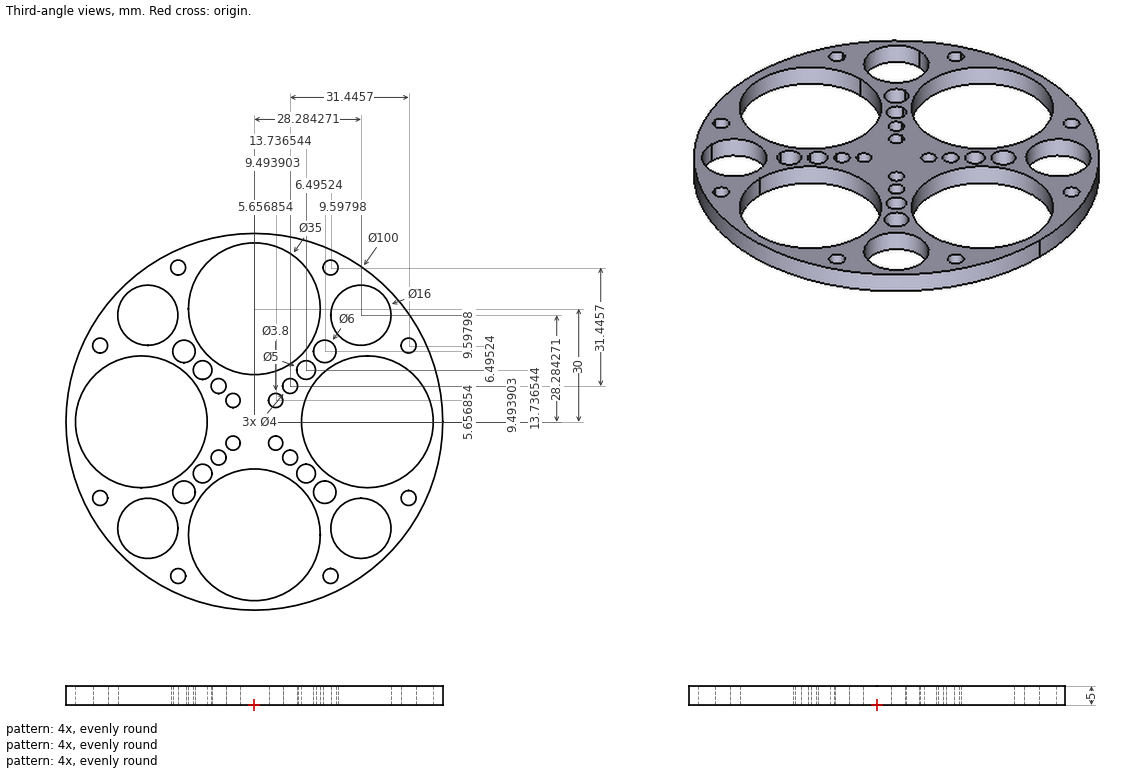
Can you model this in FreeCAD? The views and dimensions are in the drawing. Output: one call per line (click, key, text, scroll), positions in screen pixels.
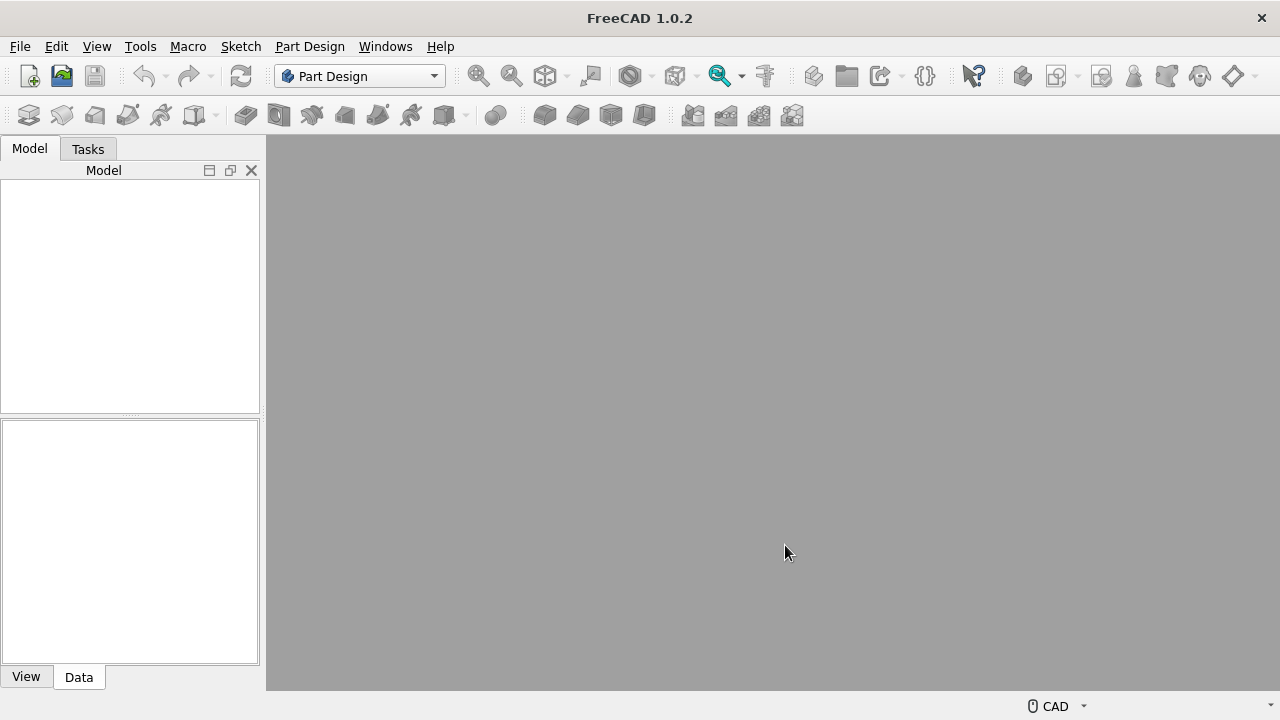
click(29, 76)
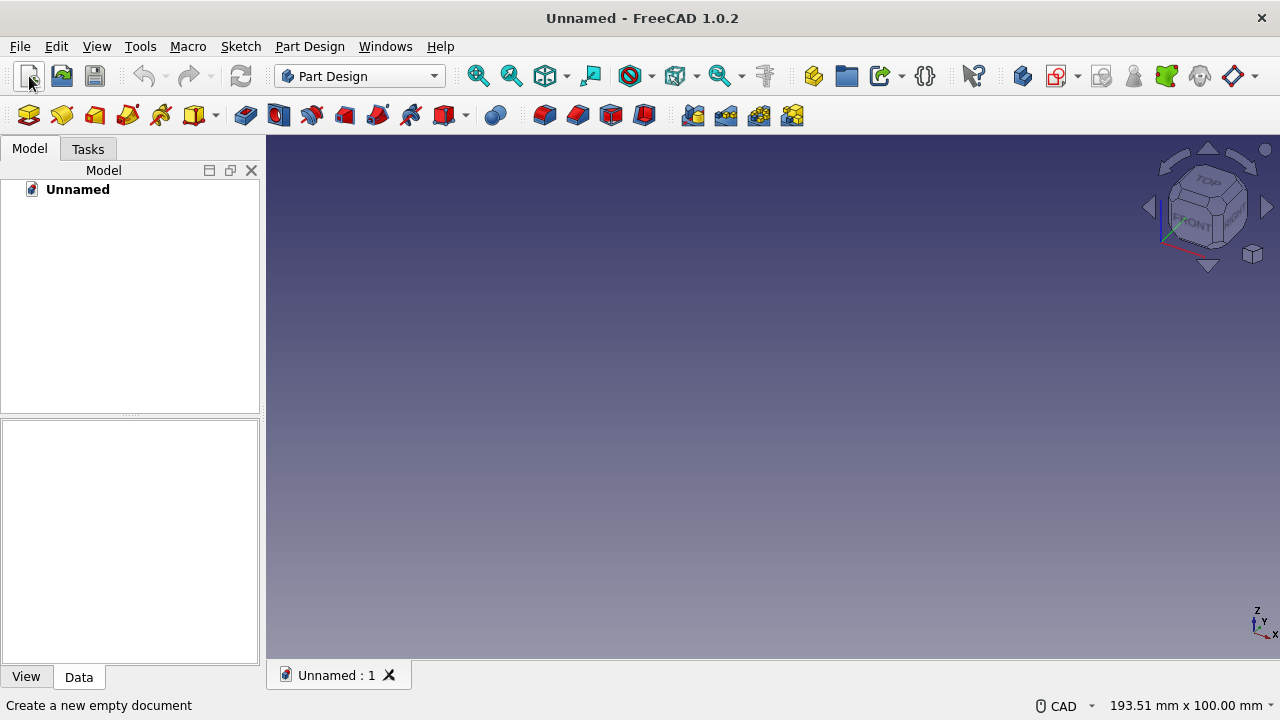
click(1056, 76)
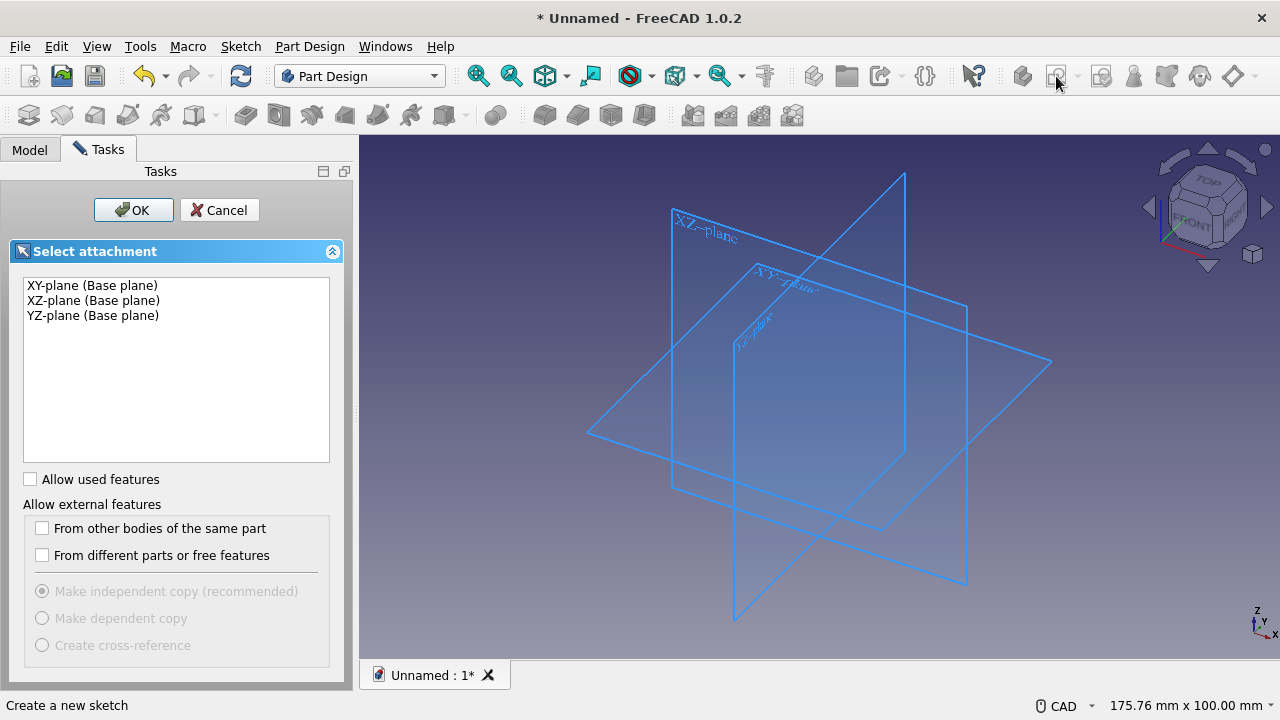
click(84, 286)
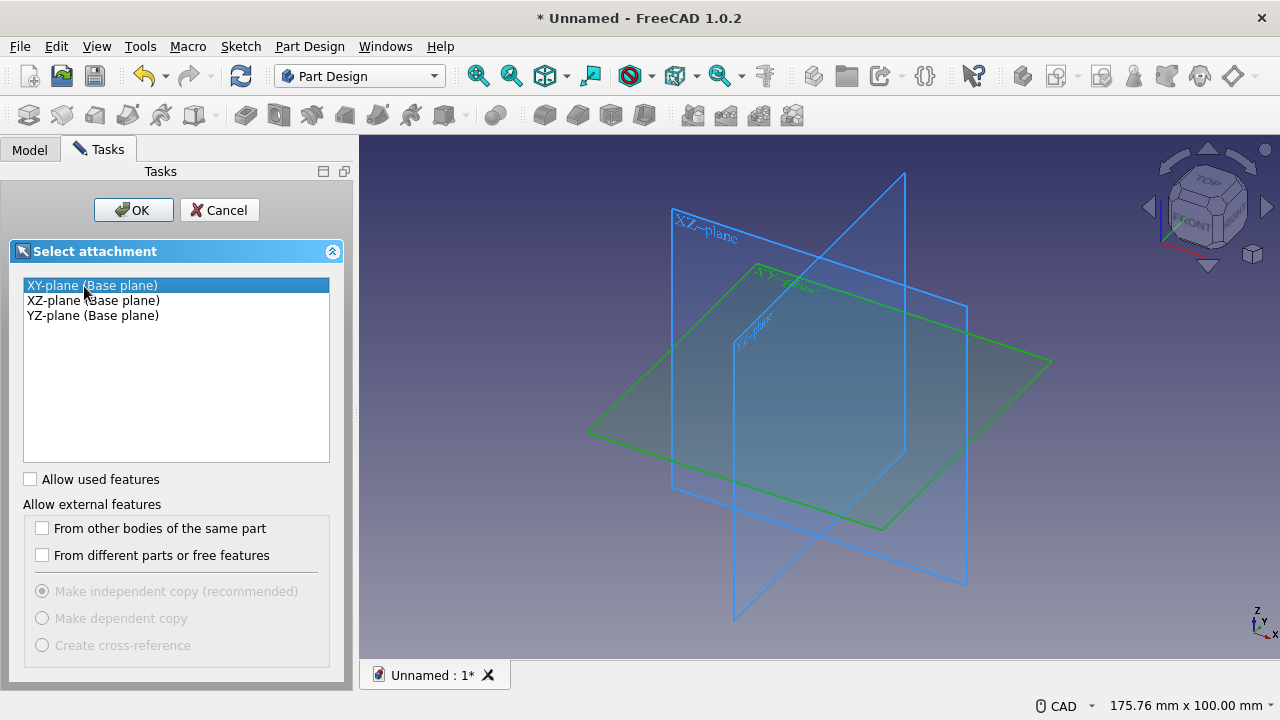
click(134, 210)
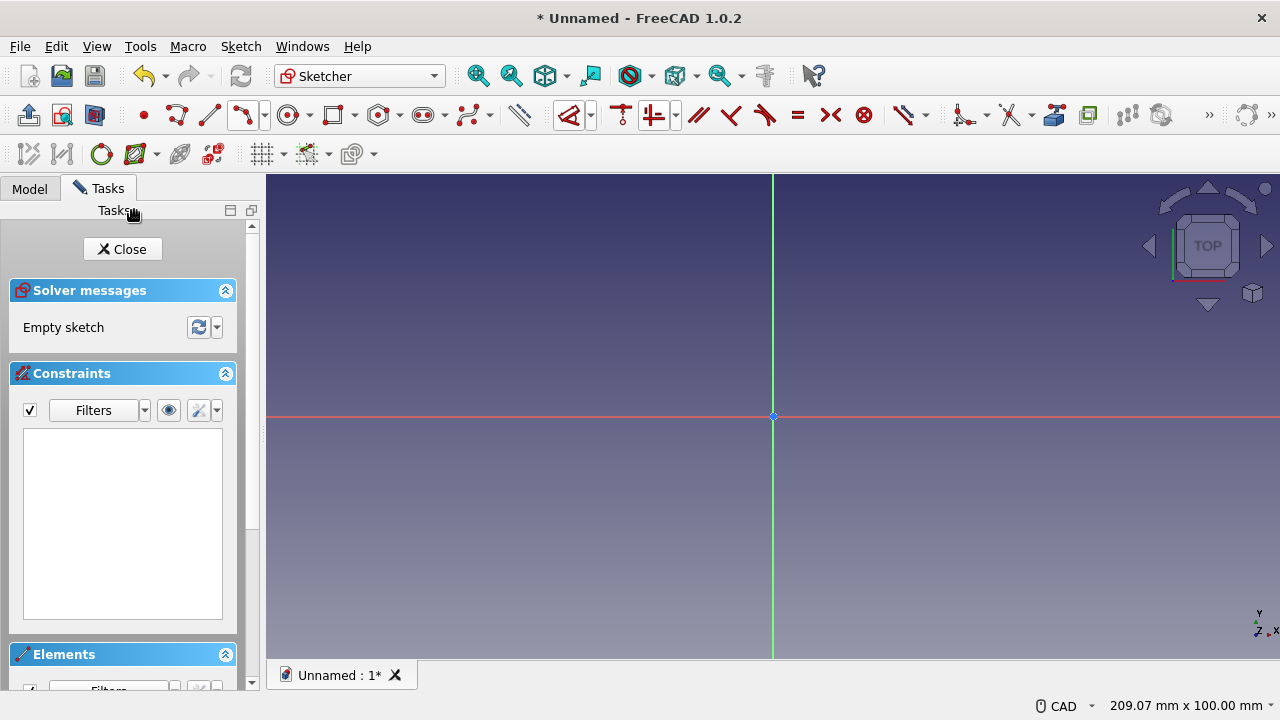
scroll(565, 416, down, 2)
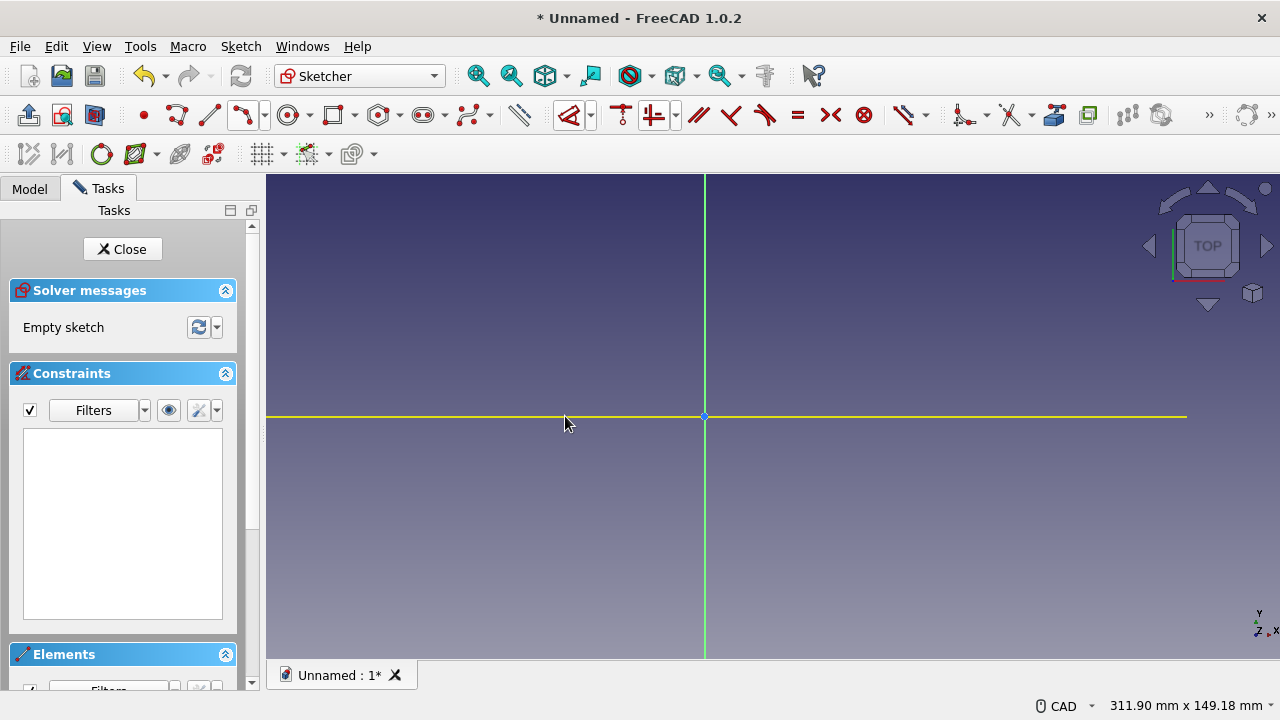
click(288, 116)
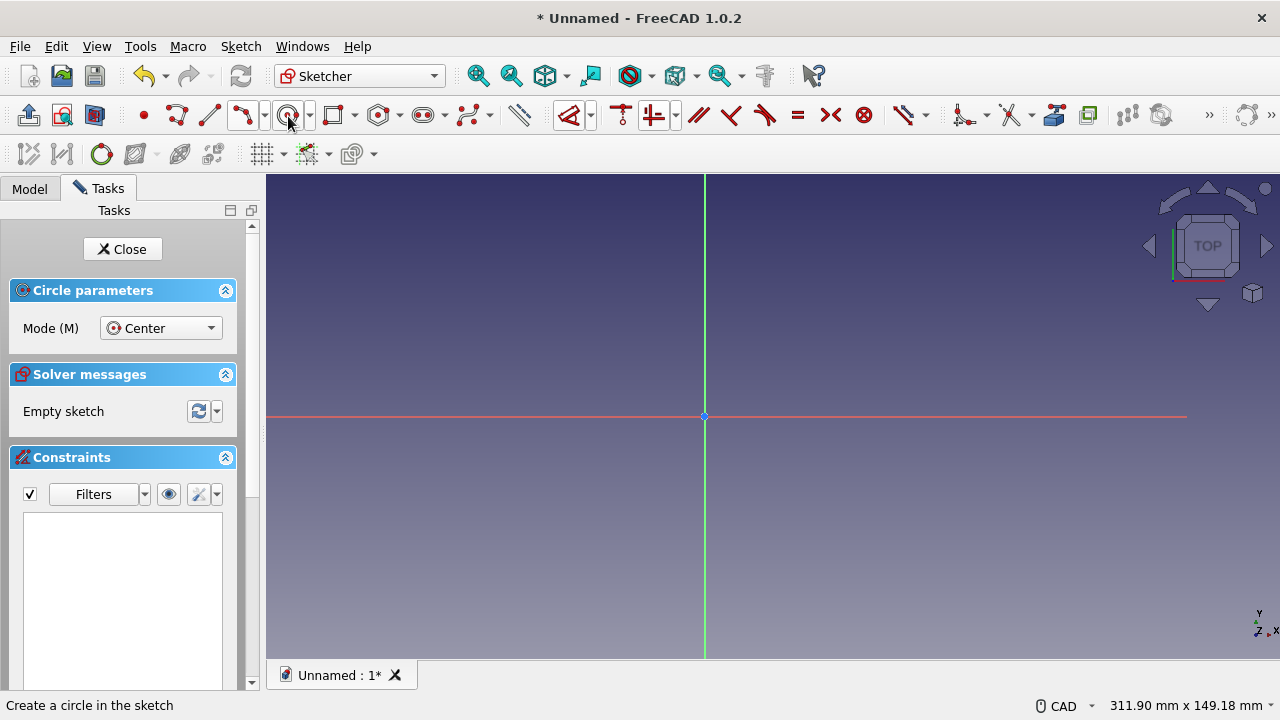
click(705, 416)
click(819, 302)
key(Escape)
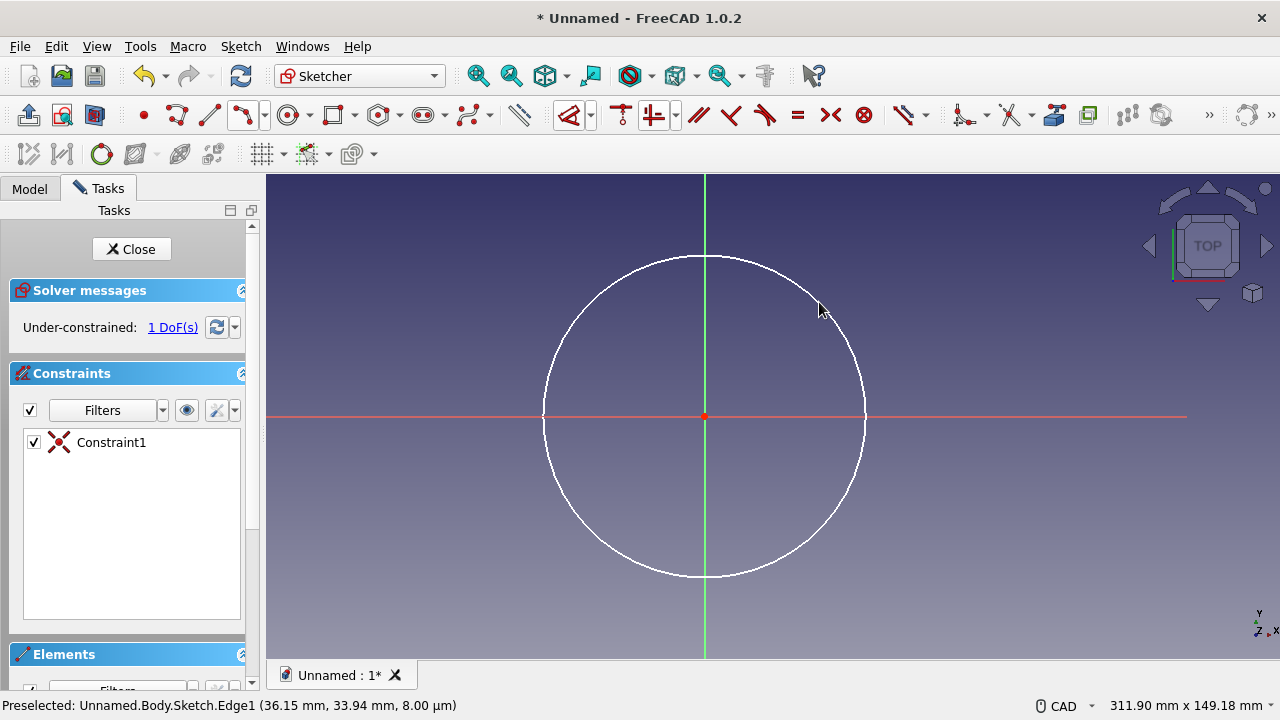
click(568, 116)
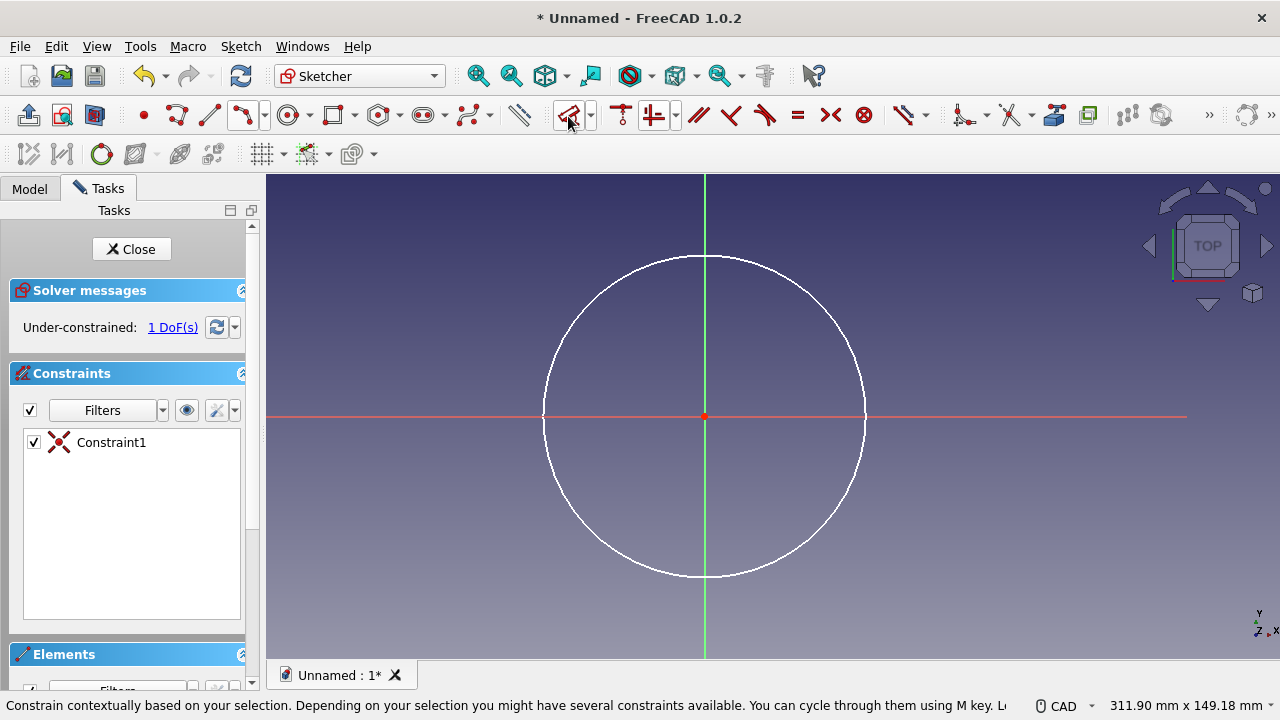
click(818, 302)
click(841, 279)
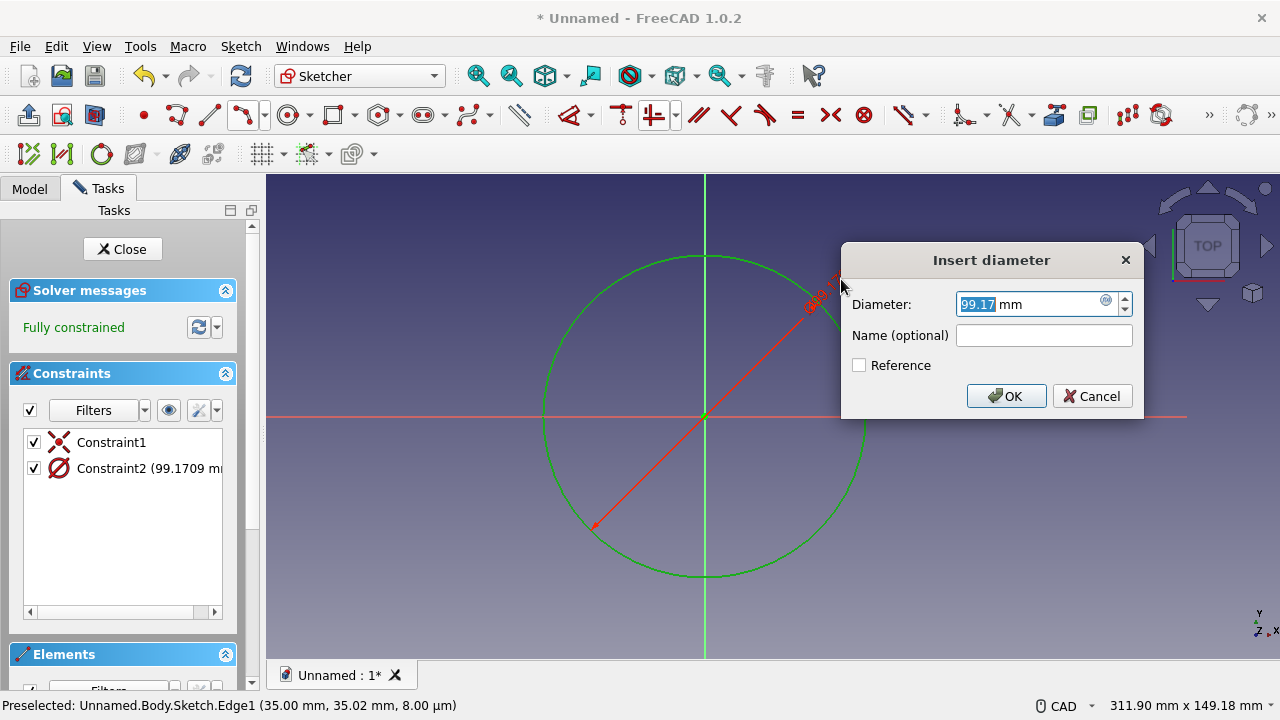
text(100)
key(Return)
key(Escape)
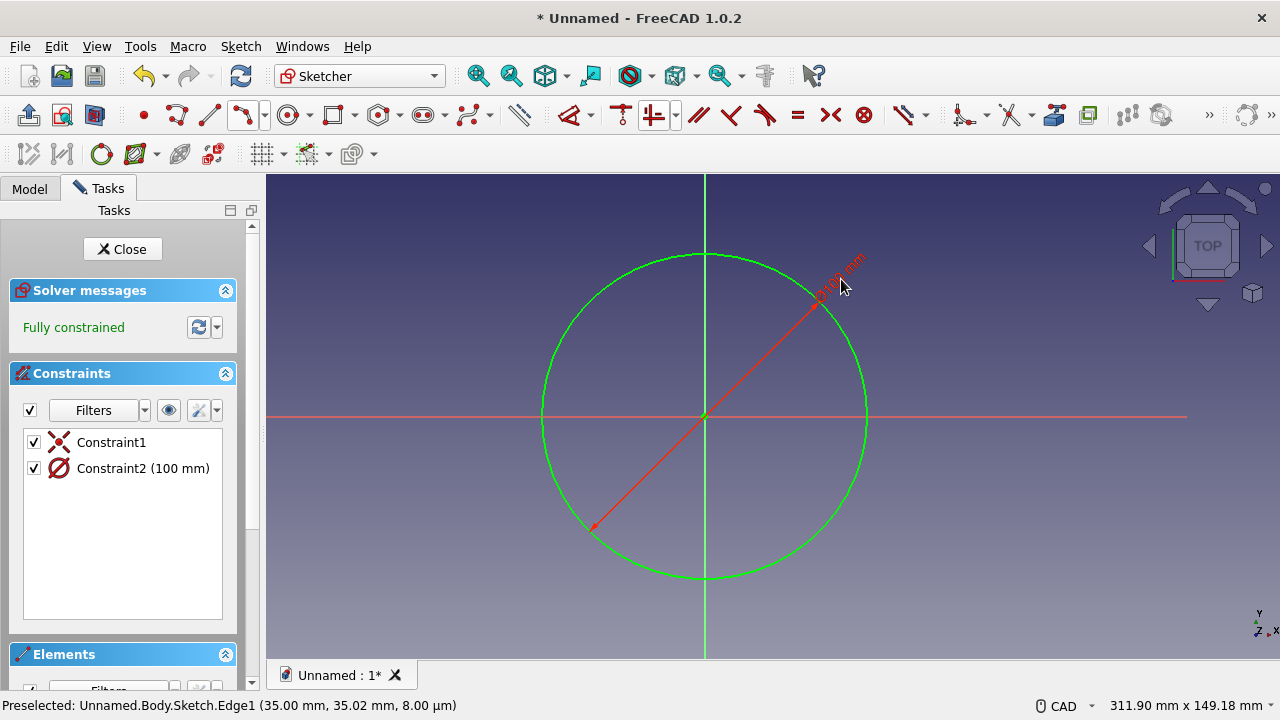
click(123, 249)